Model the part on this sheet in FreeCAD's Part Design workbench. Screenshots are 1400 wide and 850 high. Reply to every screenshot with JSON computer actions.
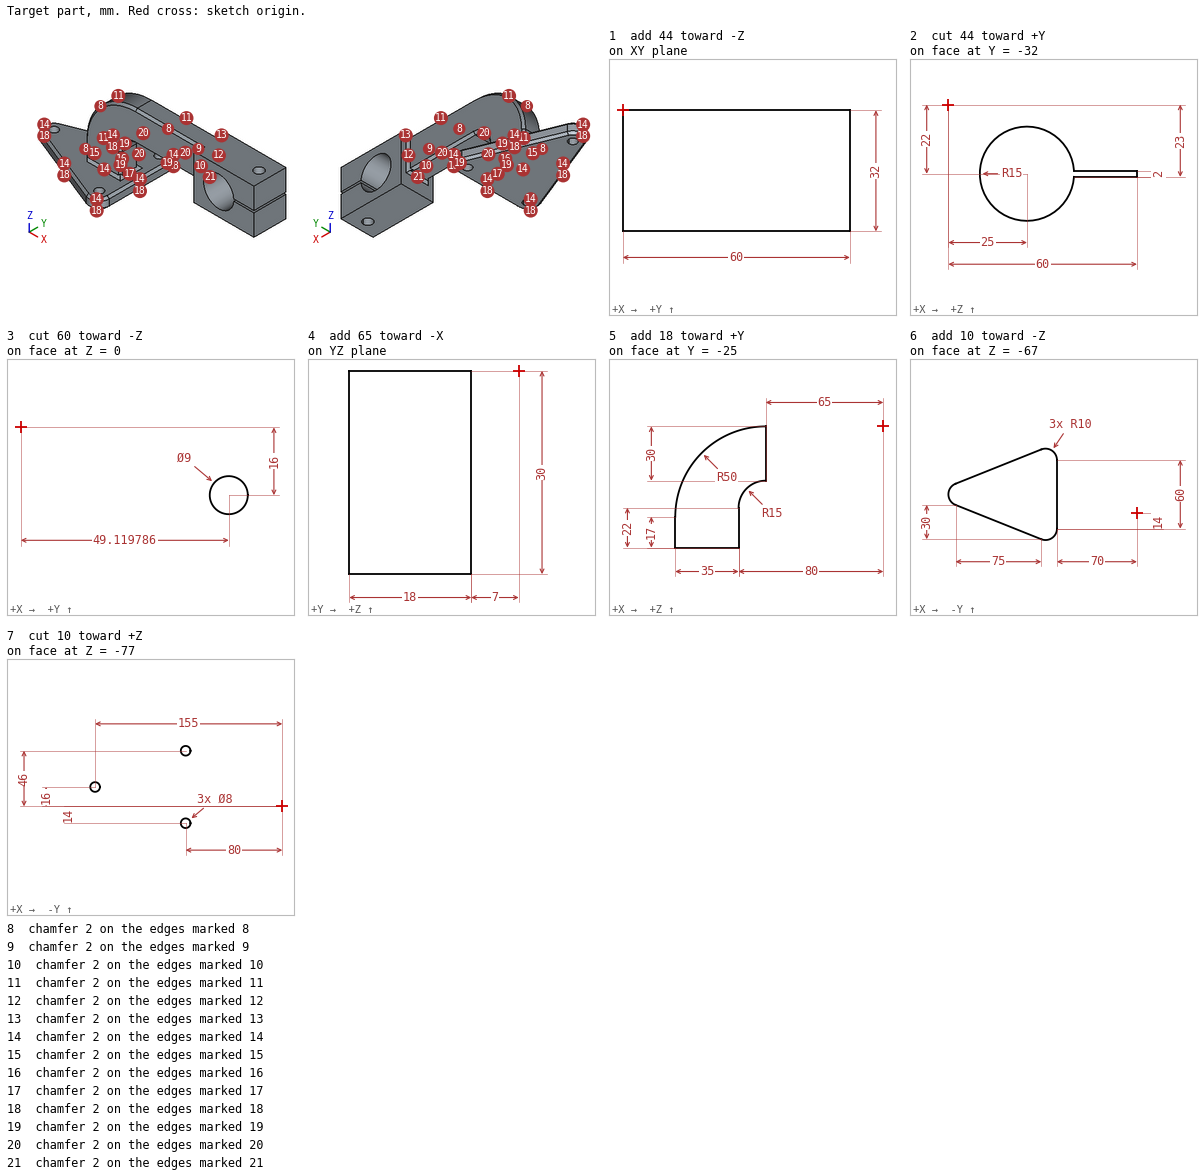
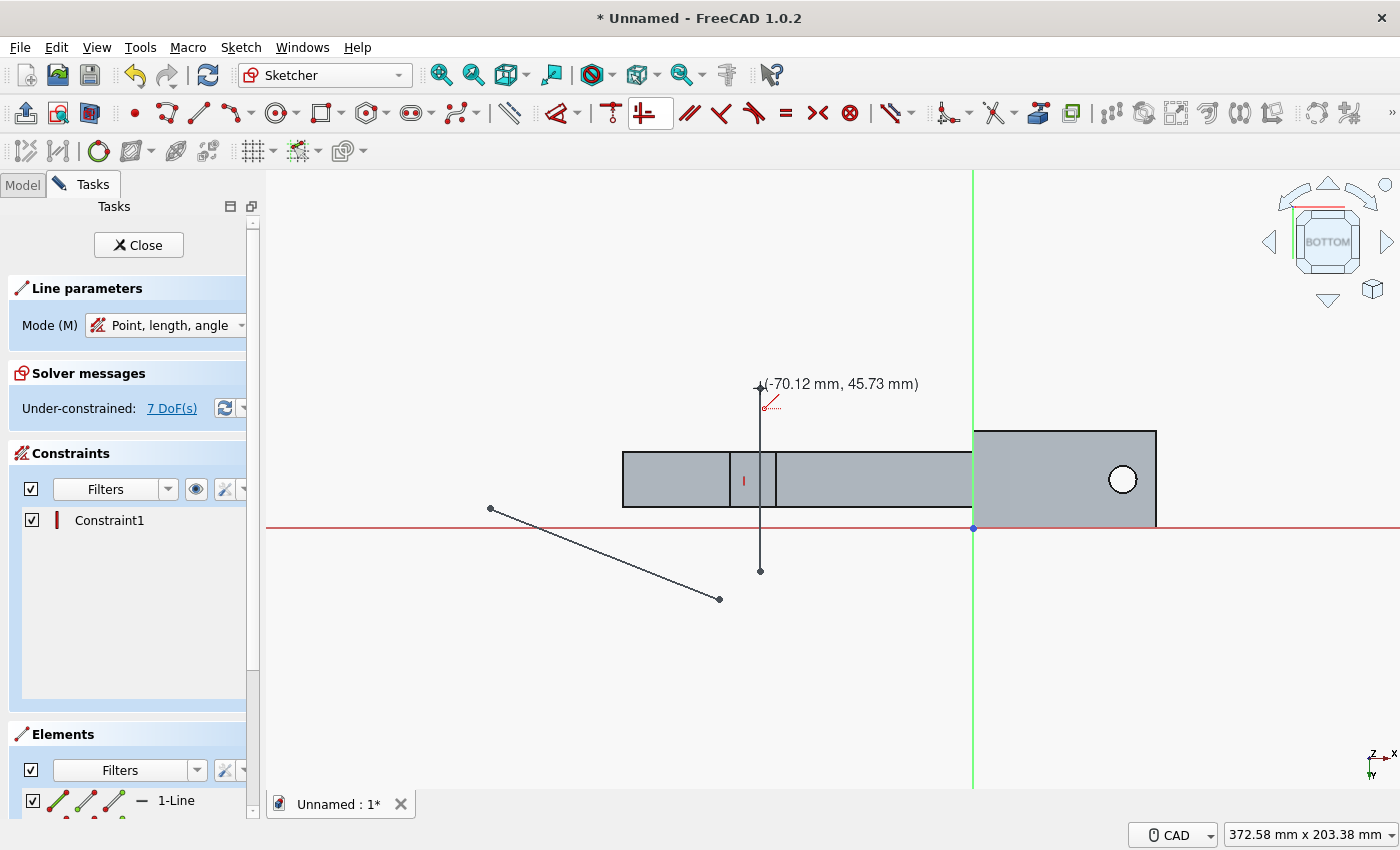
{"action": "left_click", "coordinate": [719, 360]}
{"action": "left_click", "coordinate": [490, 451]}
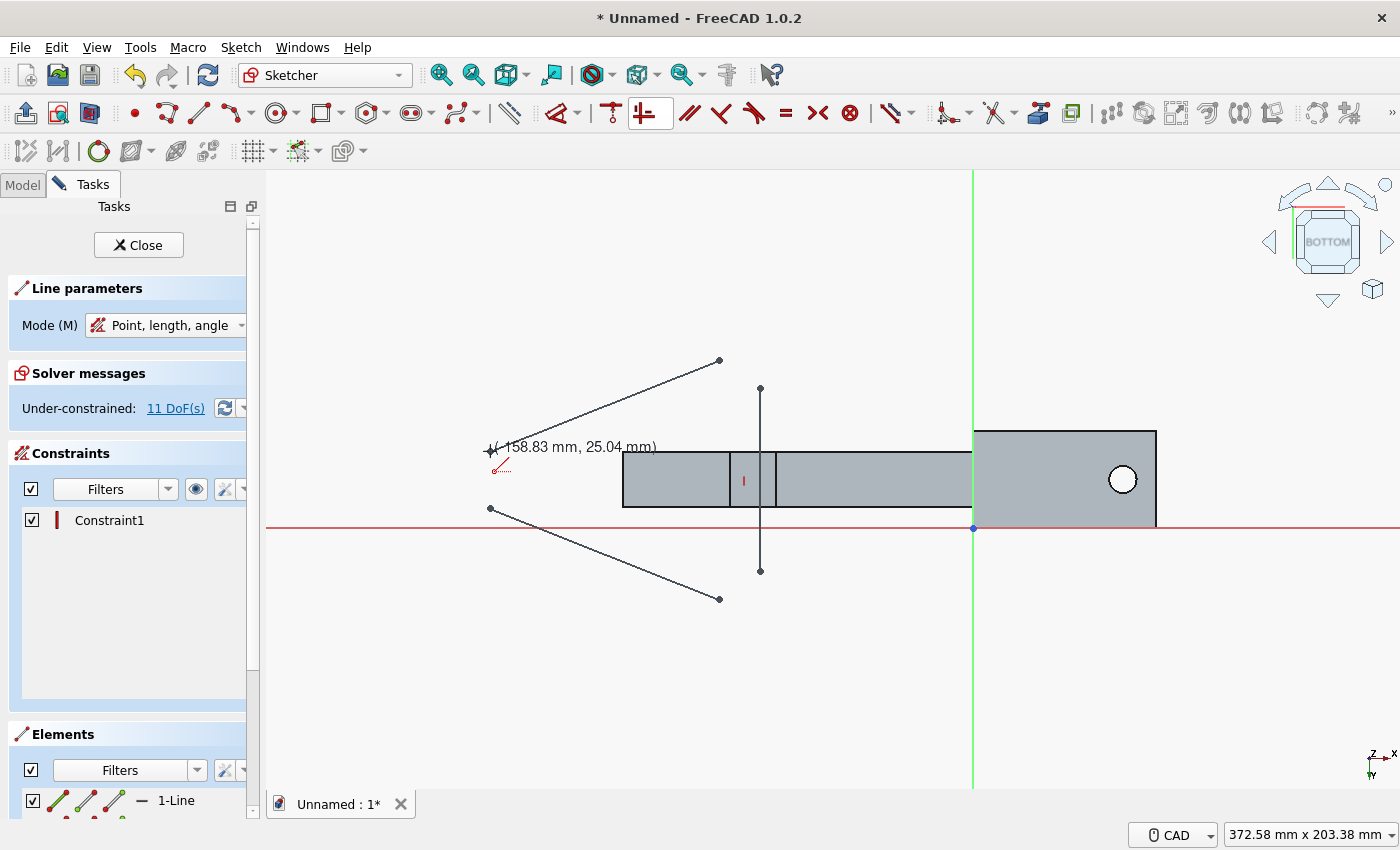
{"action": "left_click", "coordinate": [232, 114]}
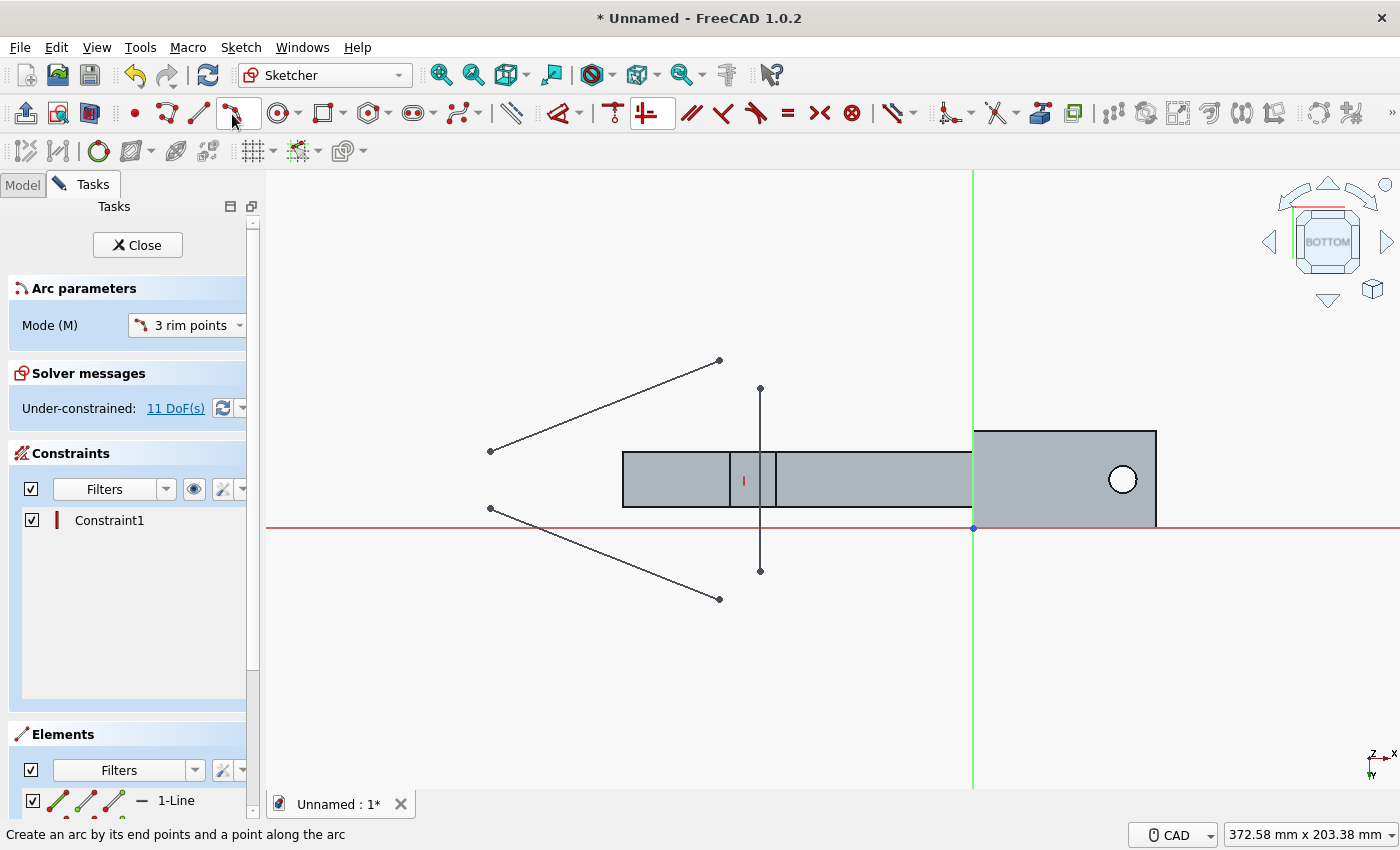
{"action": "left_click", "coordinate": [719, 600]}
{"action": "left_click", "coordinate": [760, 572]}
{"action": "left_click", "coordinate": [747, 596]}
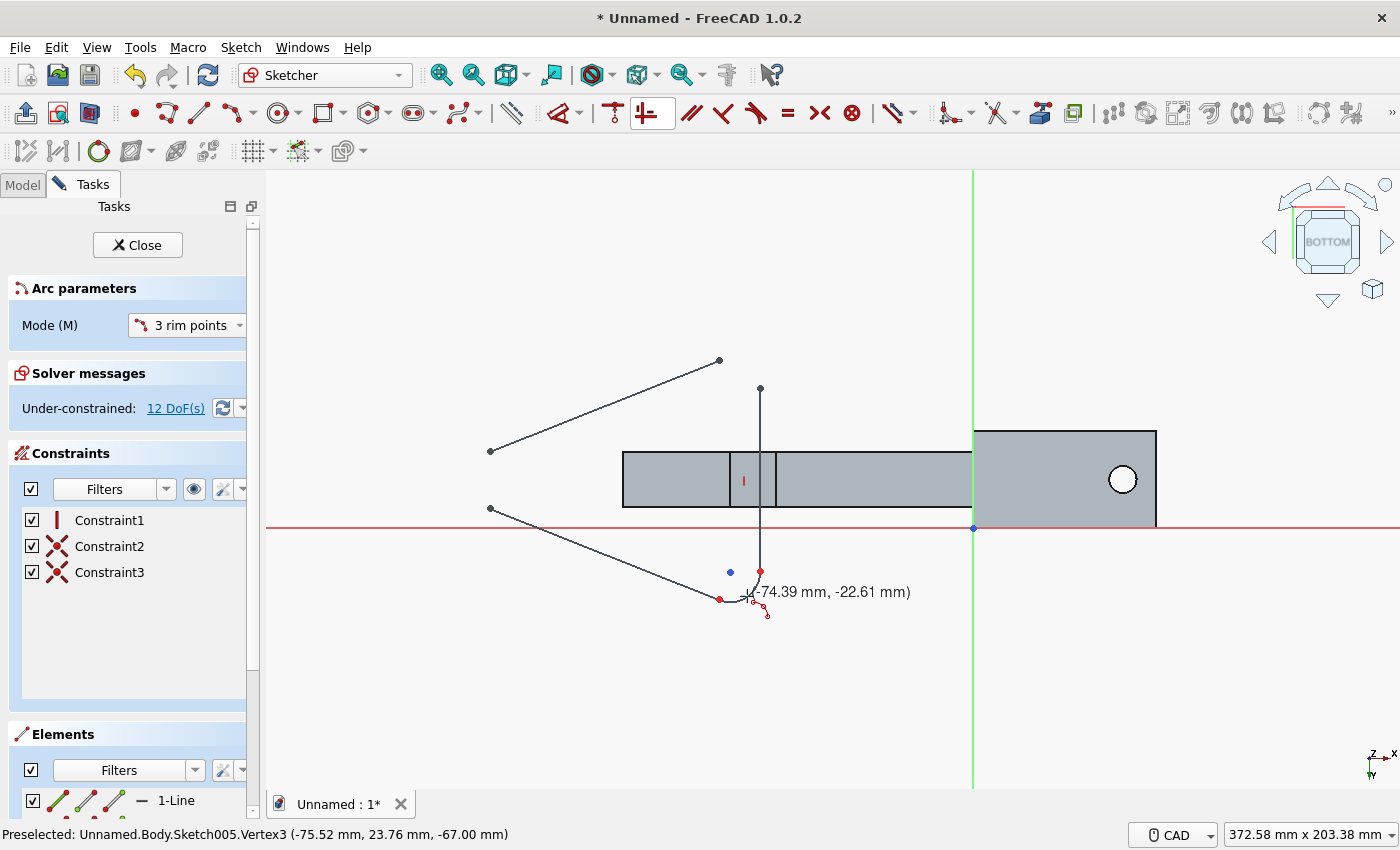
{"action": "left_click", "coordinate": [760, 389]}
{"action": "left_click", "coordinate": [719, 361]}
{"action": "left_click", "coordinate": [747, 363]}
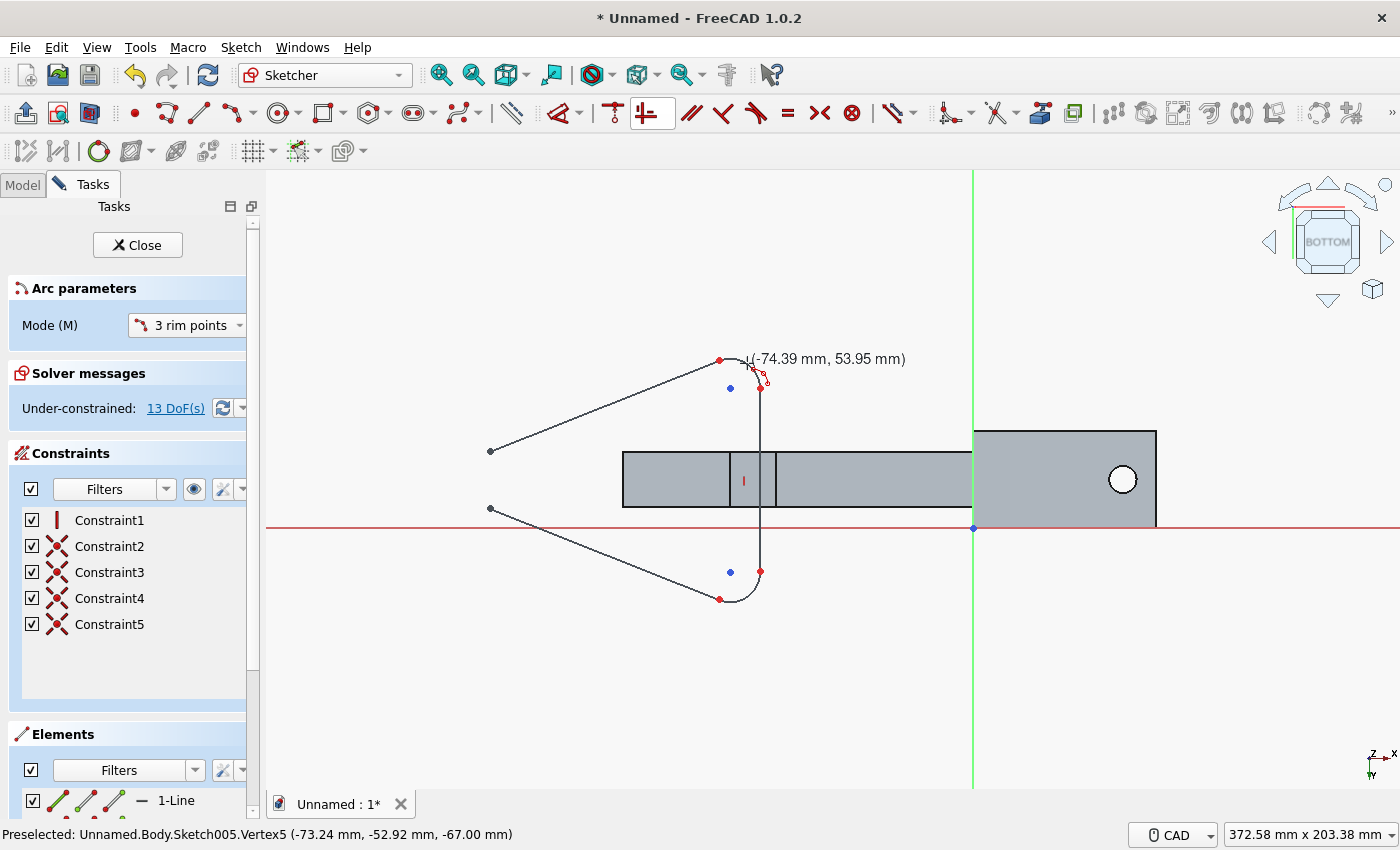
{"action": "left_click", "coordinate": [490, 452]}
{"action": "left_click", "coordinate": [490, 509]}
{"action": "left_click", "coordinate": [471, 480]}
{"action": "key", "text": "Escape"}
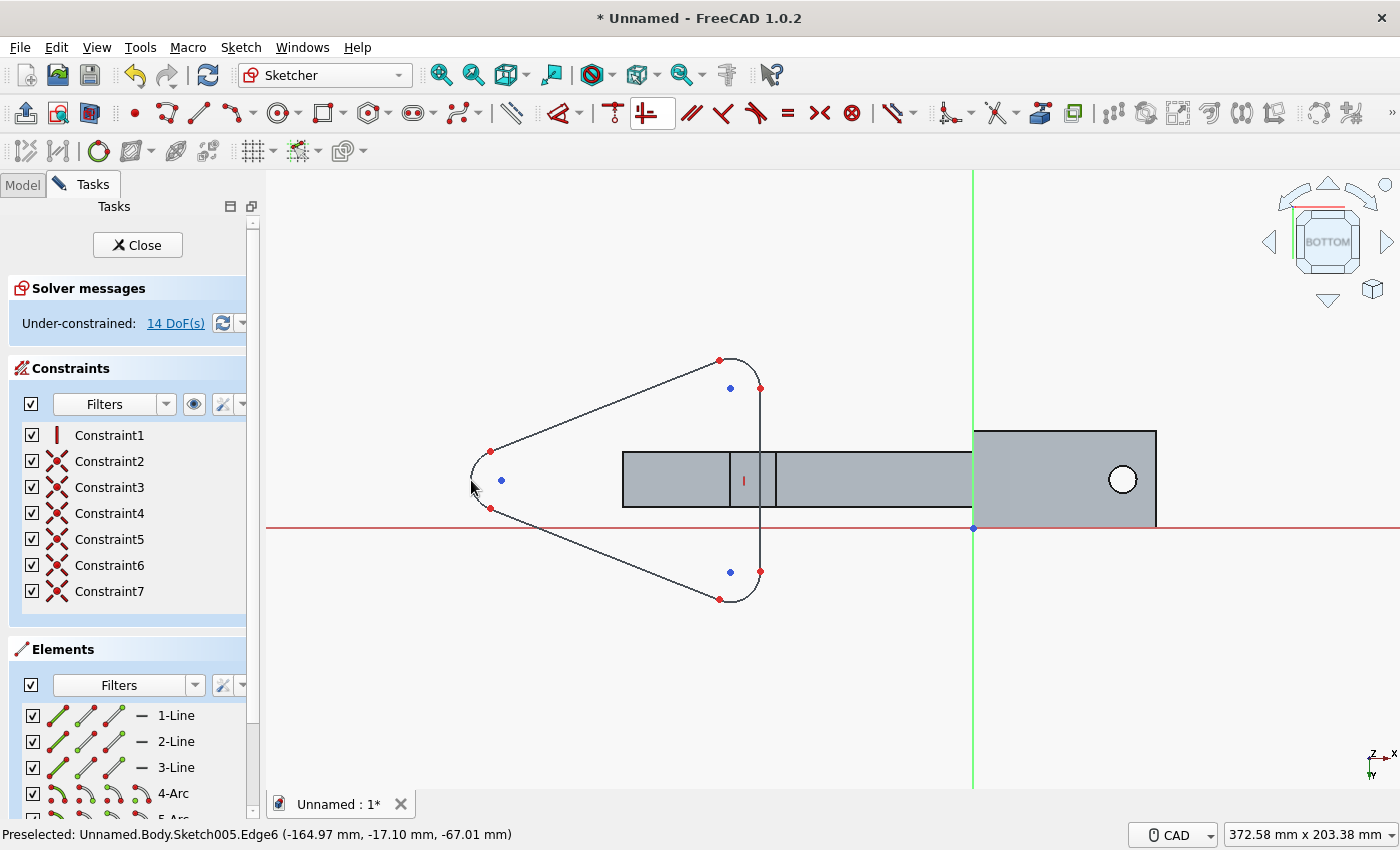
{"action": "left_click", "coordinate": [650, 573]}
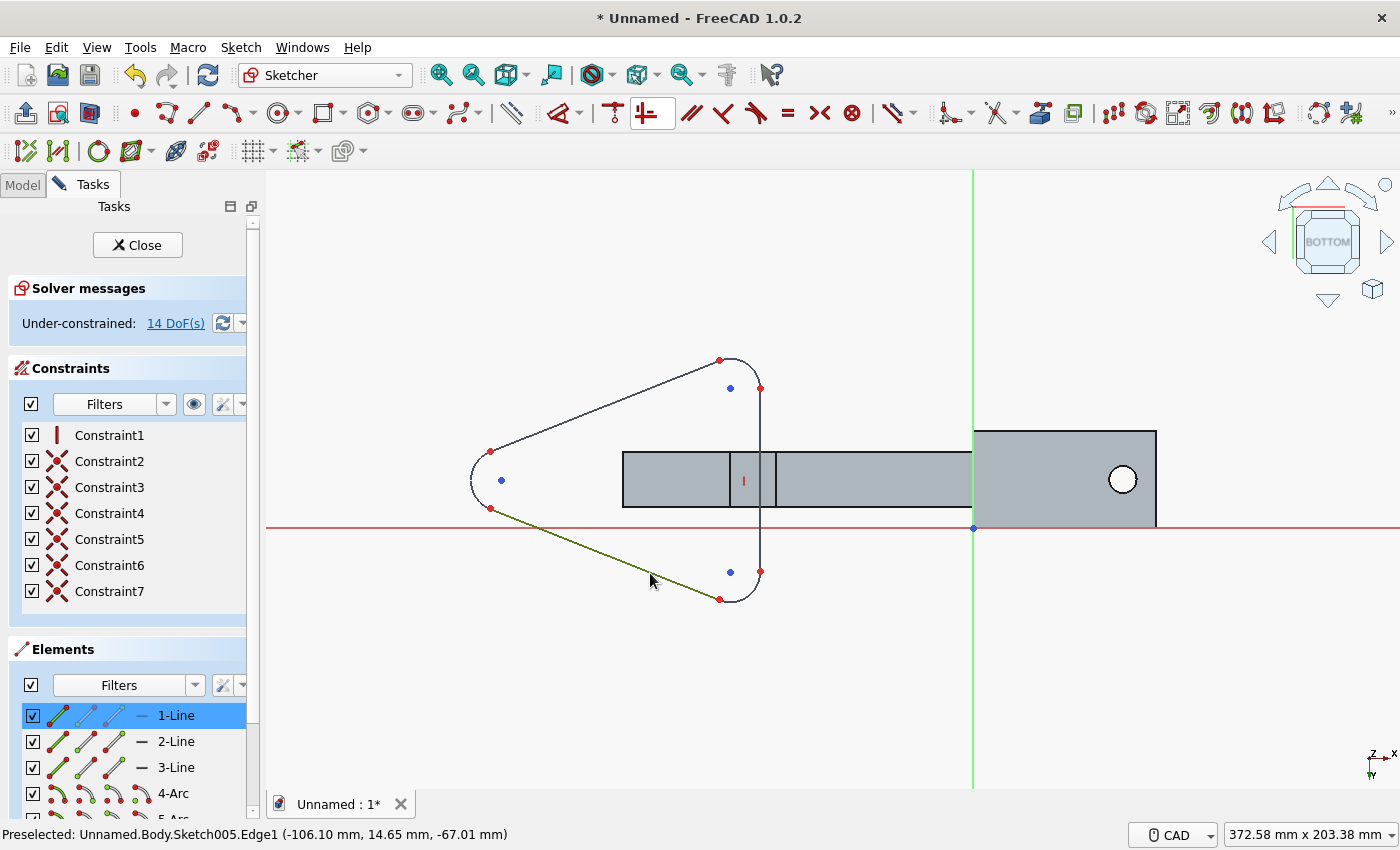
{"action": "left_click", "coordinate": [736, 602]}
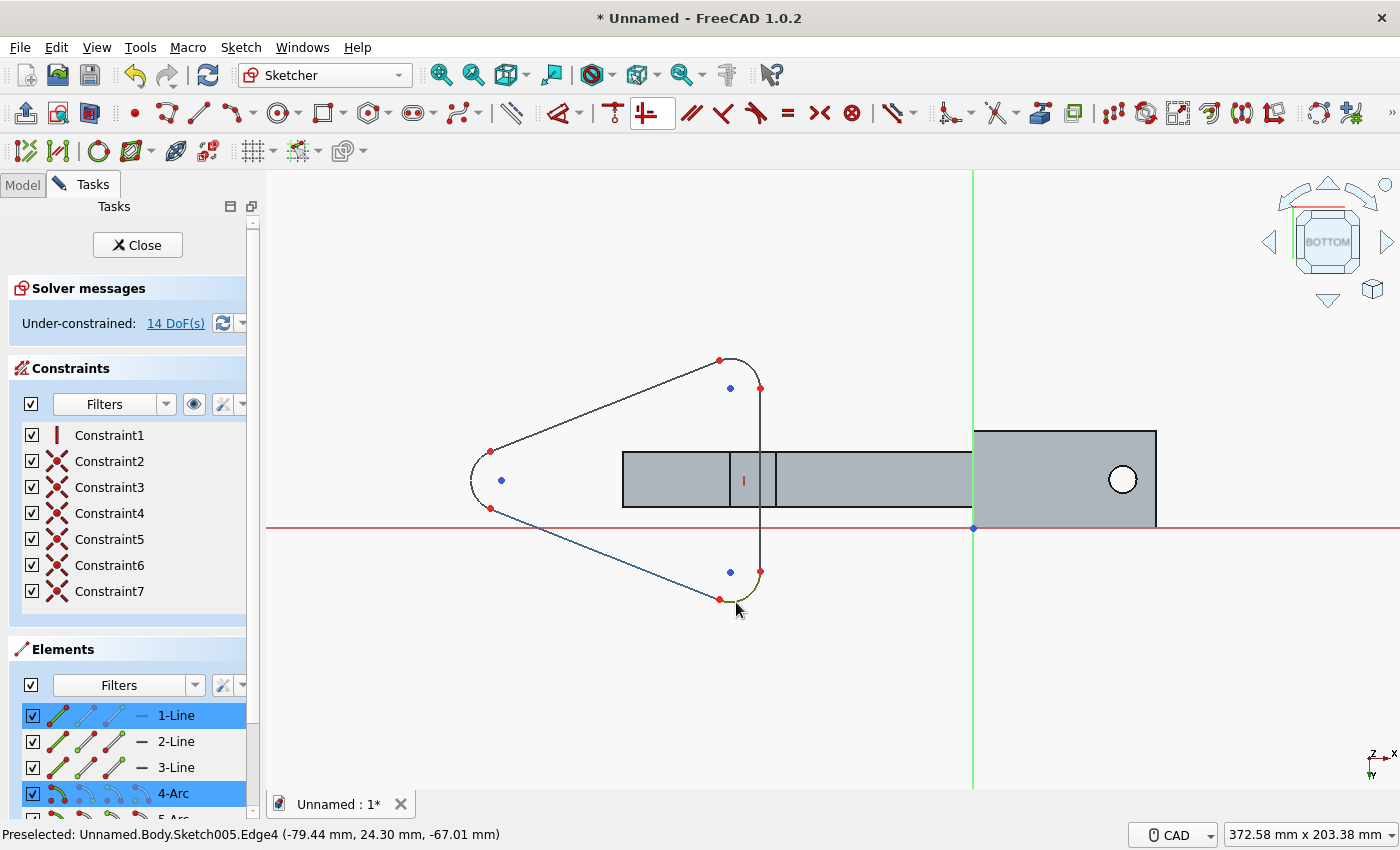
{"action": "left_click", "coordinate": [756, 114]}